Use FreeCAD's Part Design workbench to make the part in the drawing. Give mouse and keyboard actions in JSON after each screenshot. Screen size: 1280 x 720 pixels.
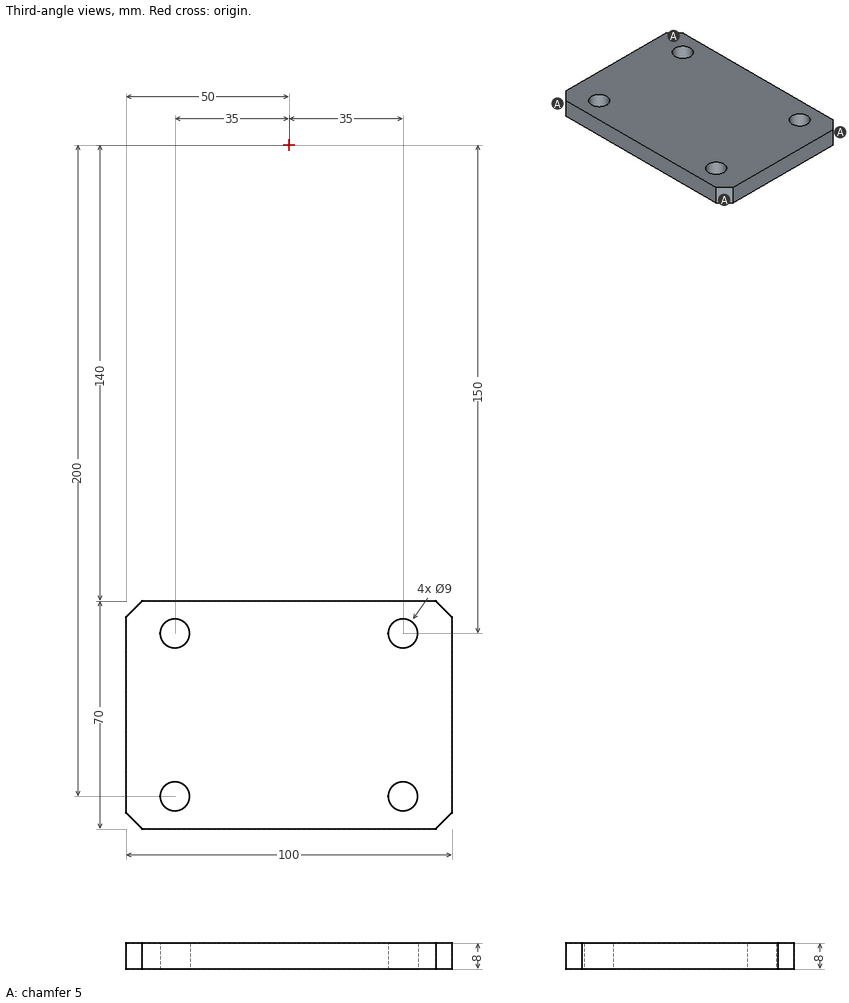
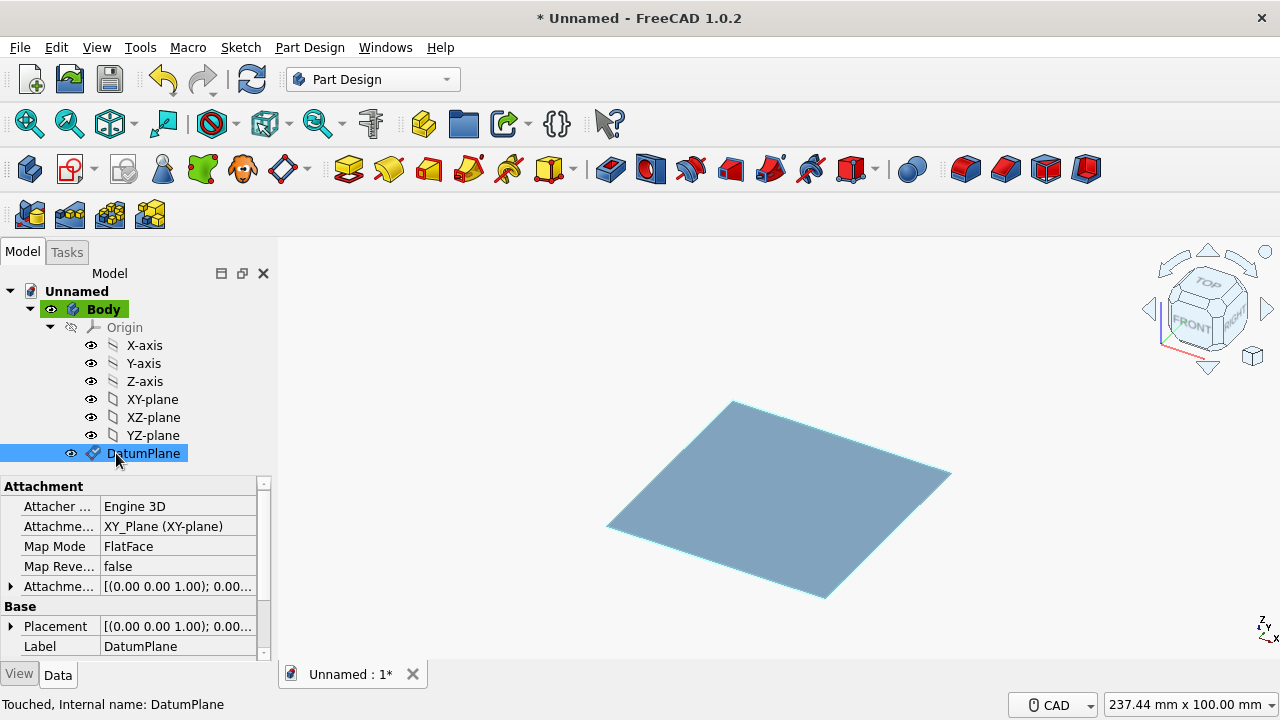
{"action": "left_click", "coordinate": [70, 170]}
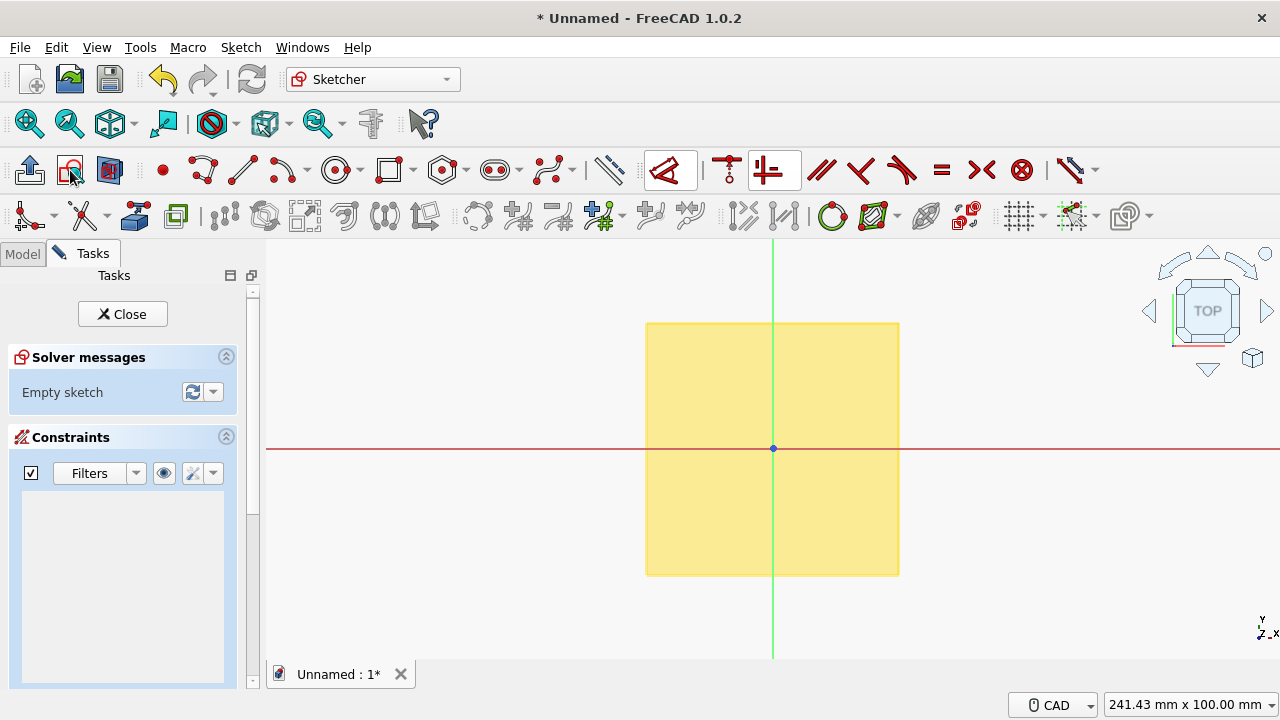
{"action": "scroll", "coordinate": [675, 267], "scroll_direction": "down", "scroll_amount": 6}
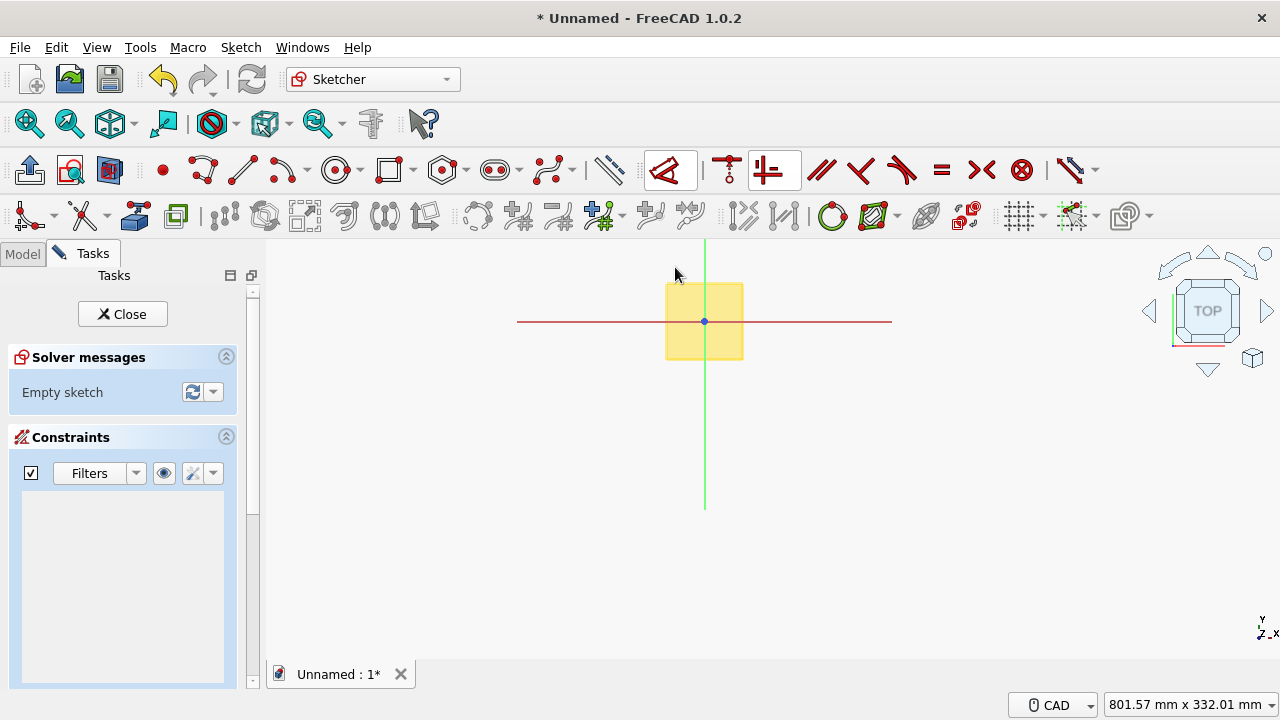
{"action": "left_click", "coordinate": [390, 170]}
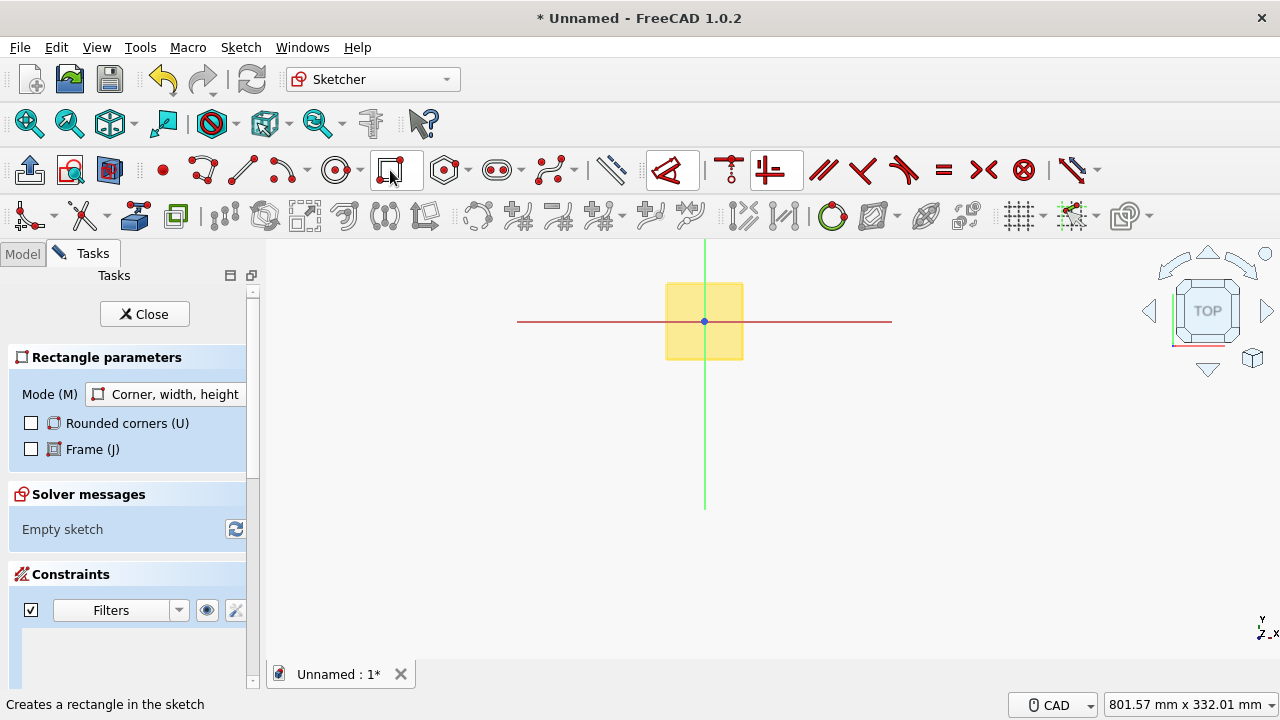
{"action": "left_click", "coordinate": [642, 499]}
{"action": "left_click", "coordinate": [768, 588]}
{"action": "key", "text": "Escape"}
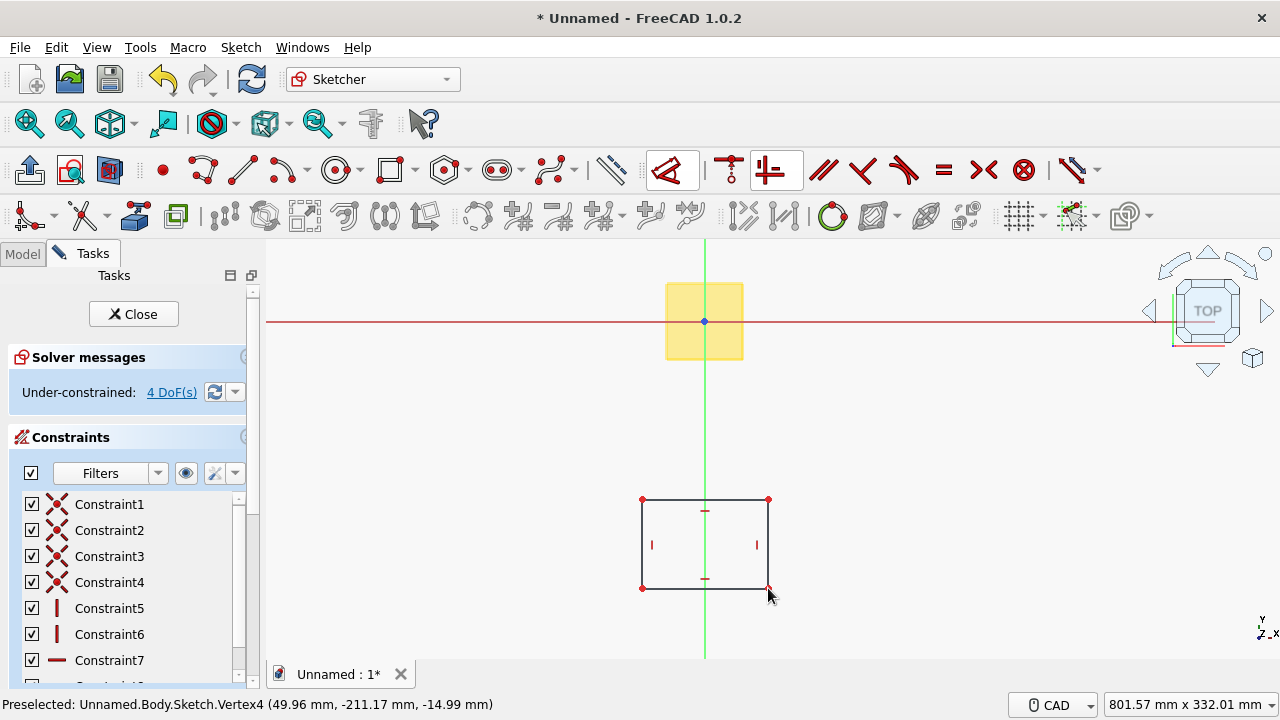
{"action": "left_click", "coordinate": [666, 170]}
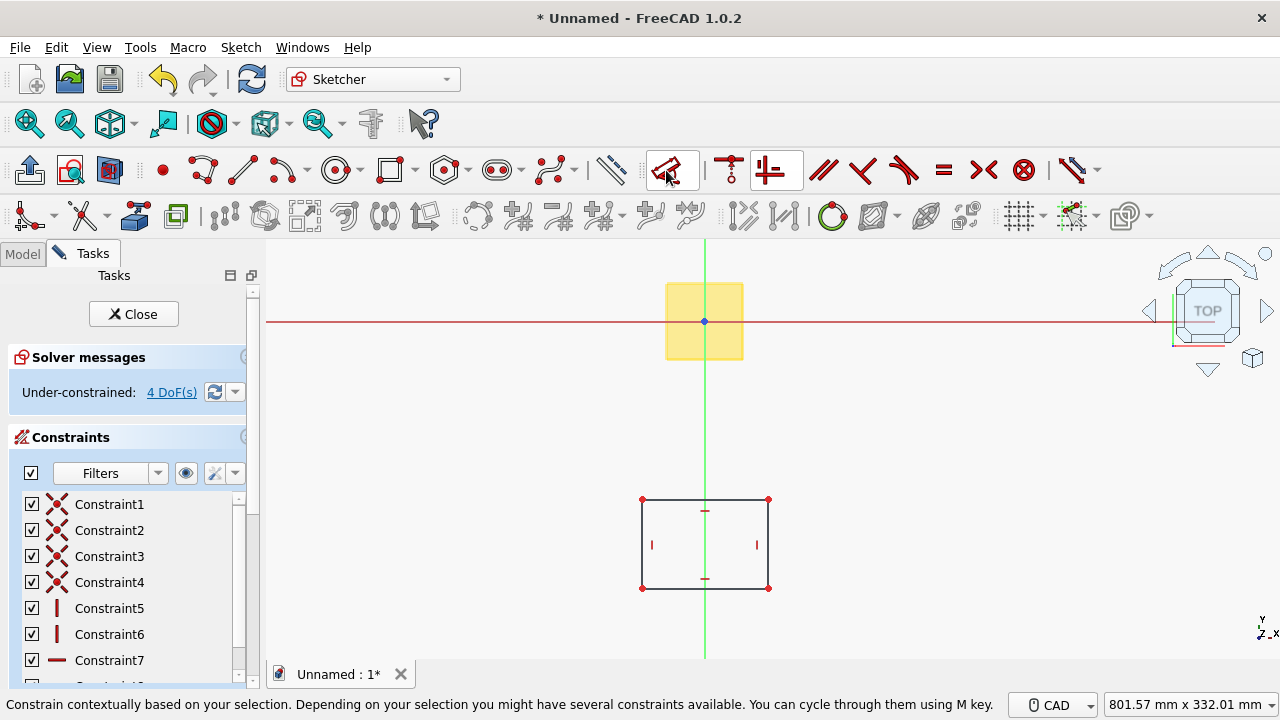
{"action": "left_click", "coordinate": [642, 527]}
{"action": "left_click", "coordinate": [608, 544]}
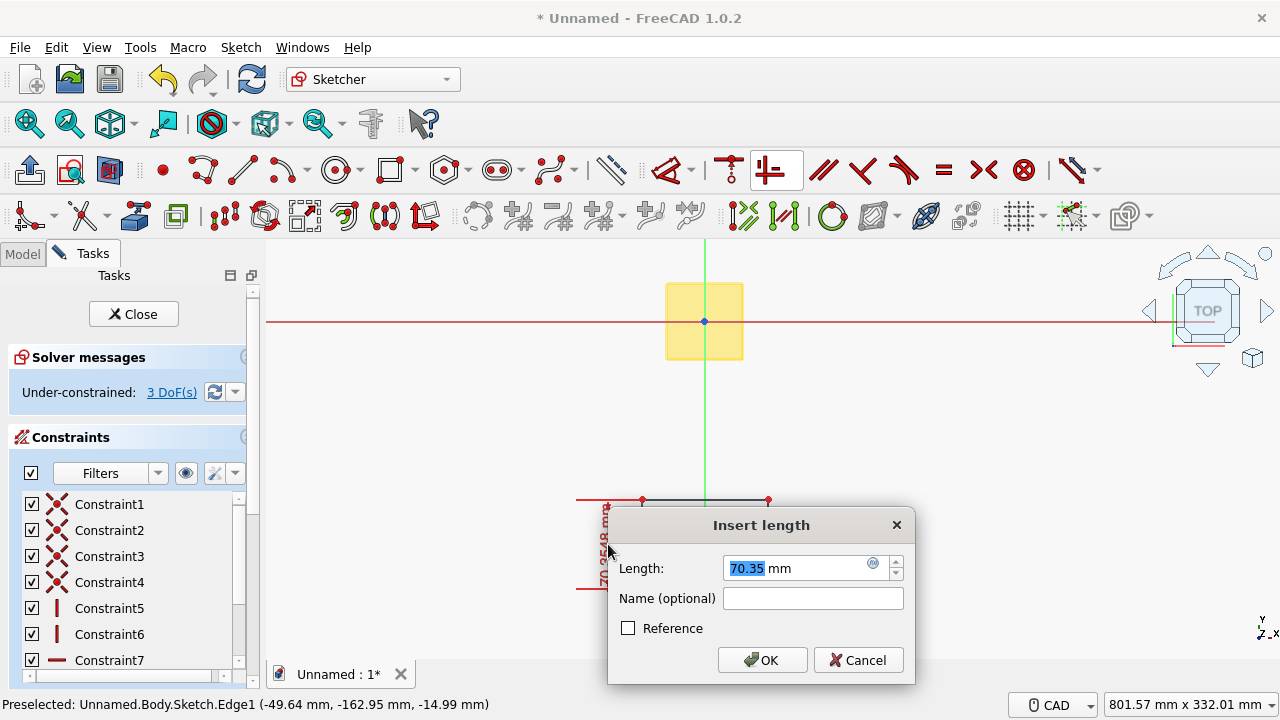
{"action": "type", "text": "70"}
{"action": "key", "text": "Return"}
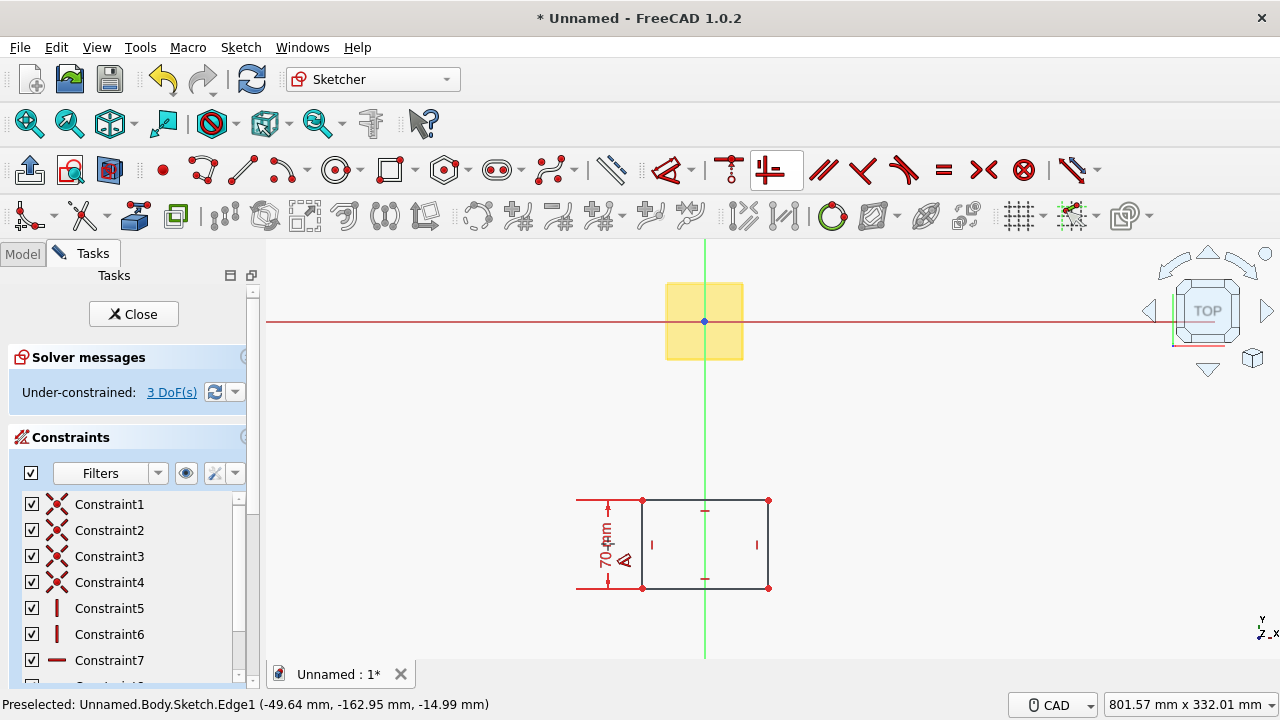
{"action": "left_click", "coordinate": [680, 589]}
{"action": "left_click", "coordinate": [676, 623]}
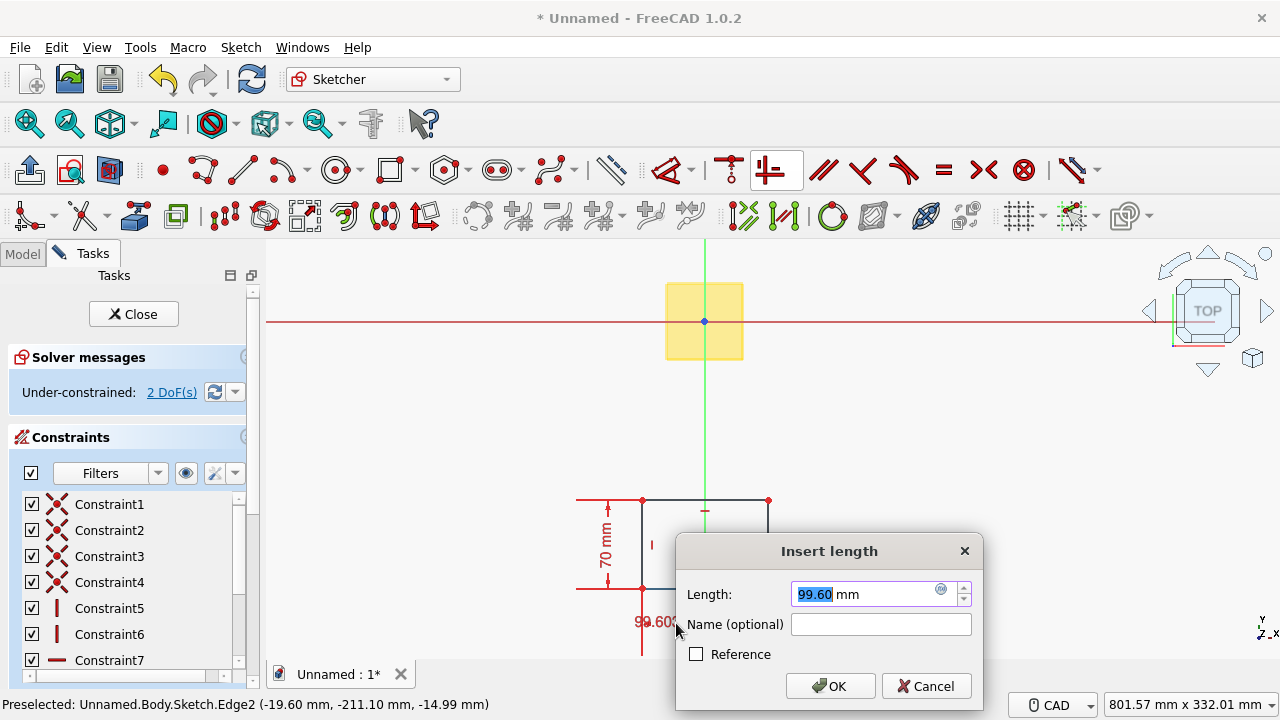
{"action": "type", "text": "100"}
{"action": "key", "text": "Return"}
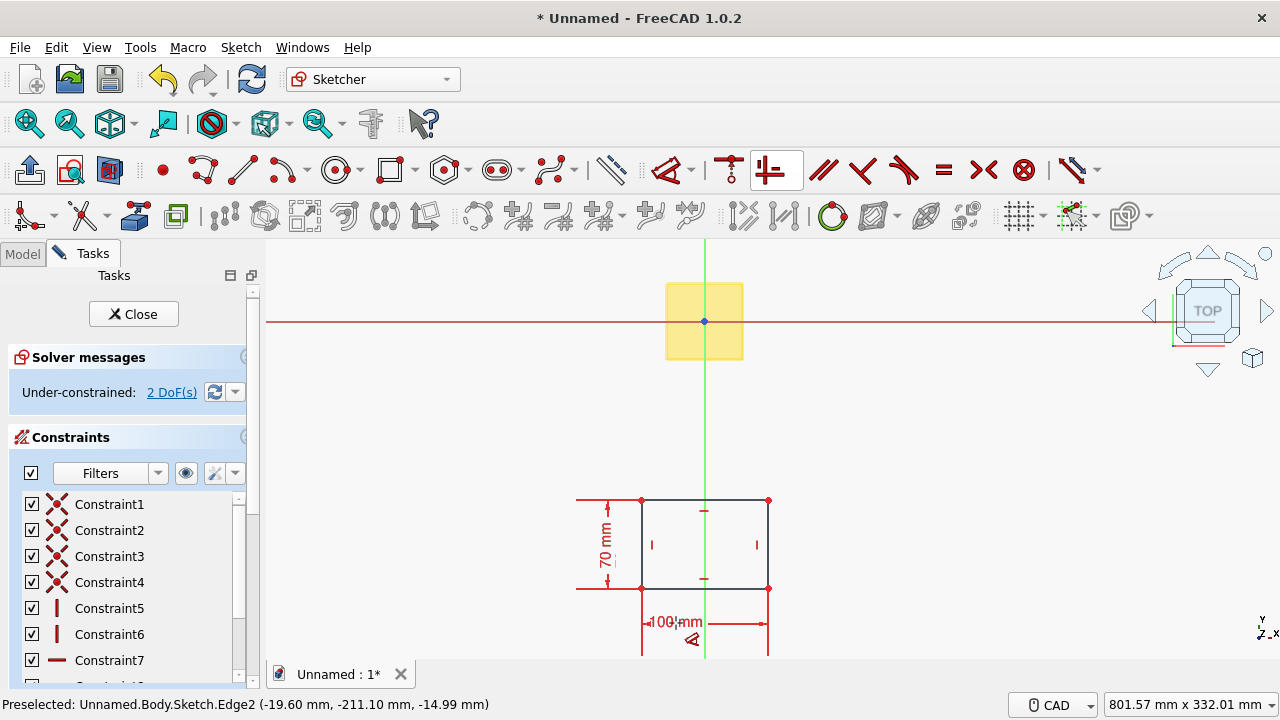
{"action": "left_click", "coordinate": [642, 500]}
{"action": "left_click", "coordinate": [673, 288]}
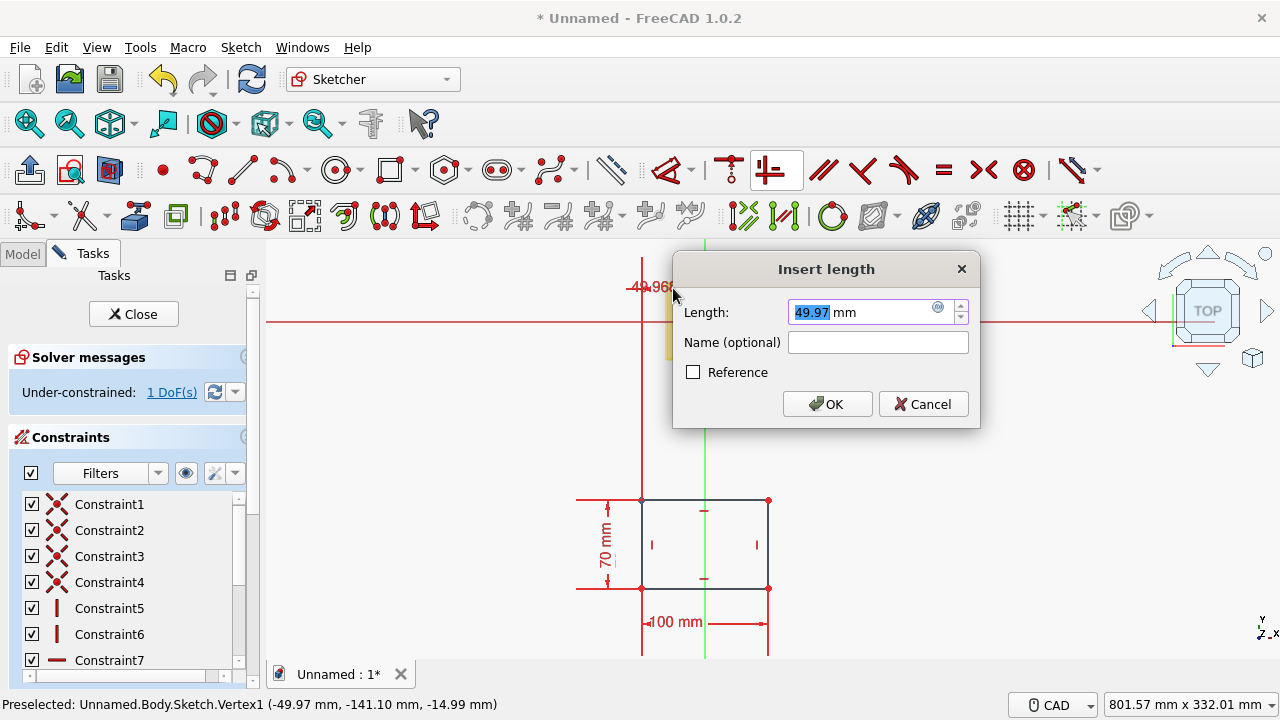
{"action": "type", "text": "50"}
{"action": "key", "text": "Return"}